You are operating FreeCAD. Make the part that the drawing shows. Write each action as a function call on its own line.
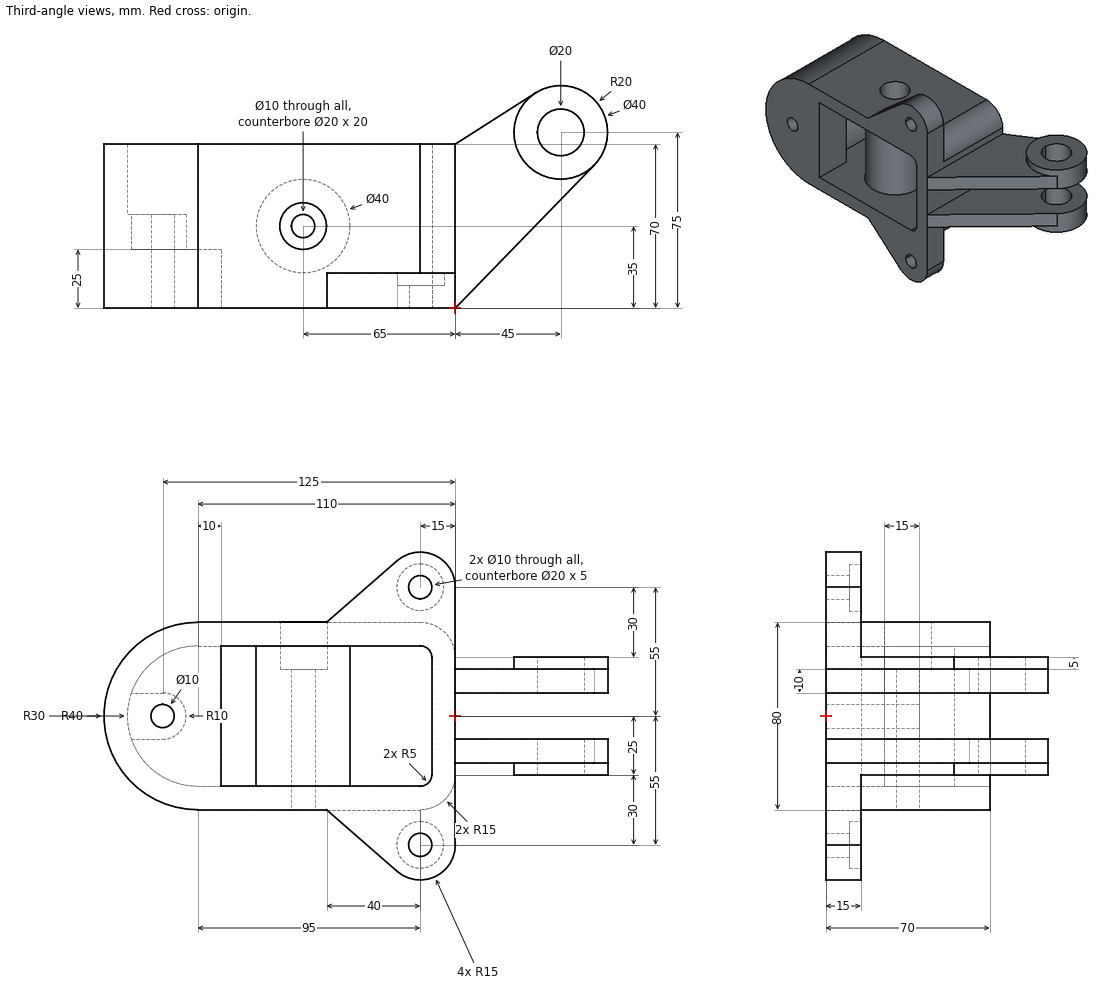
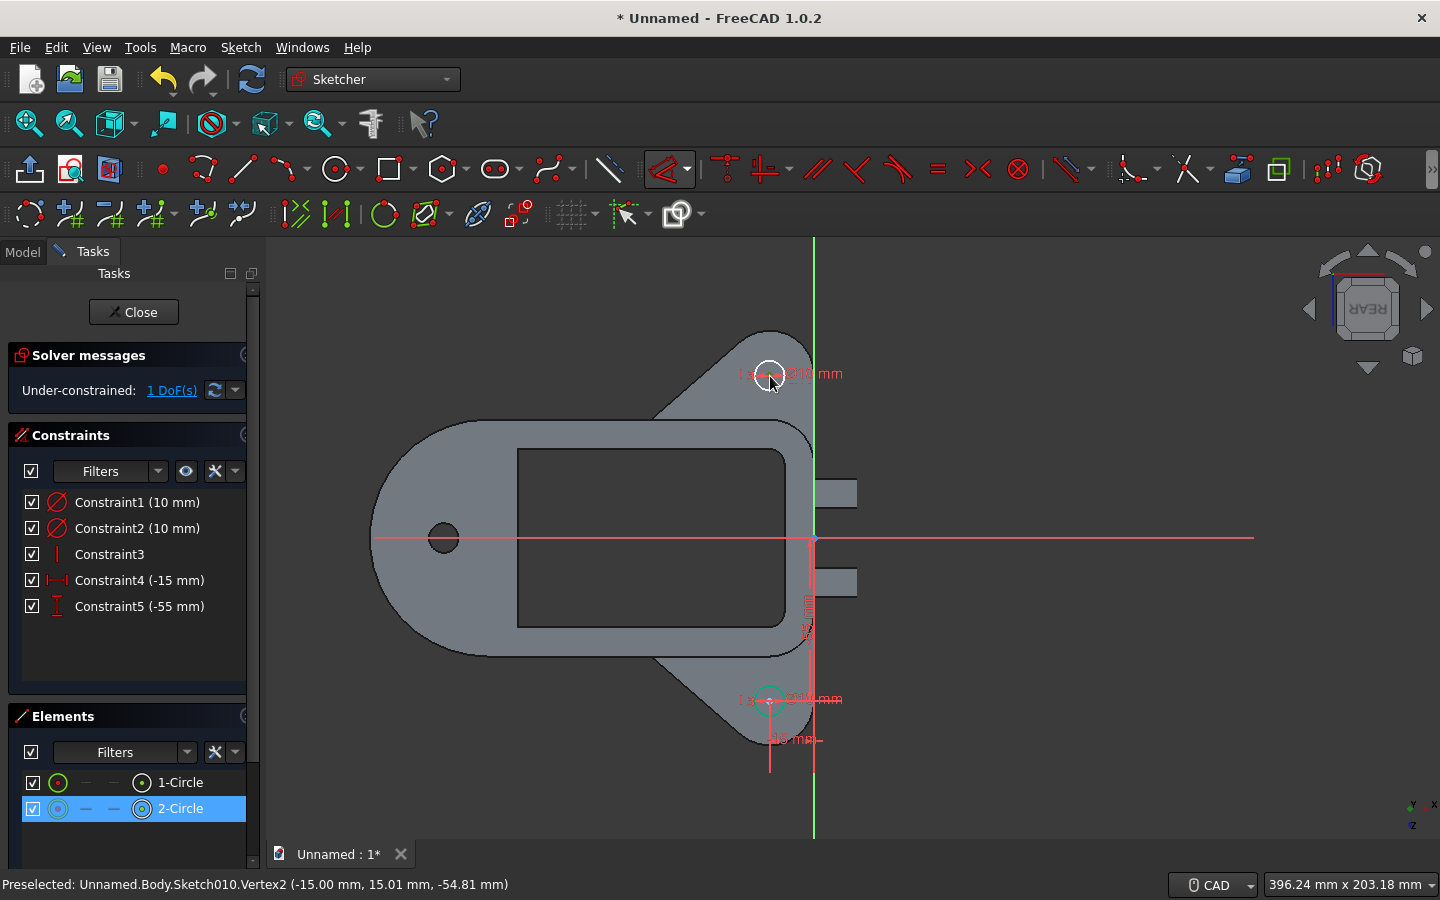
key(i)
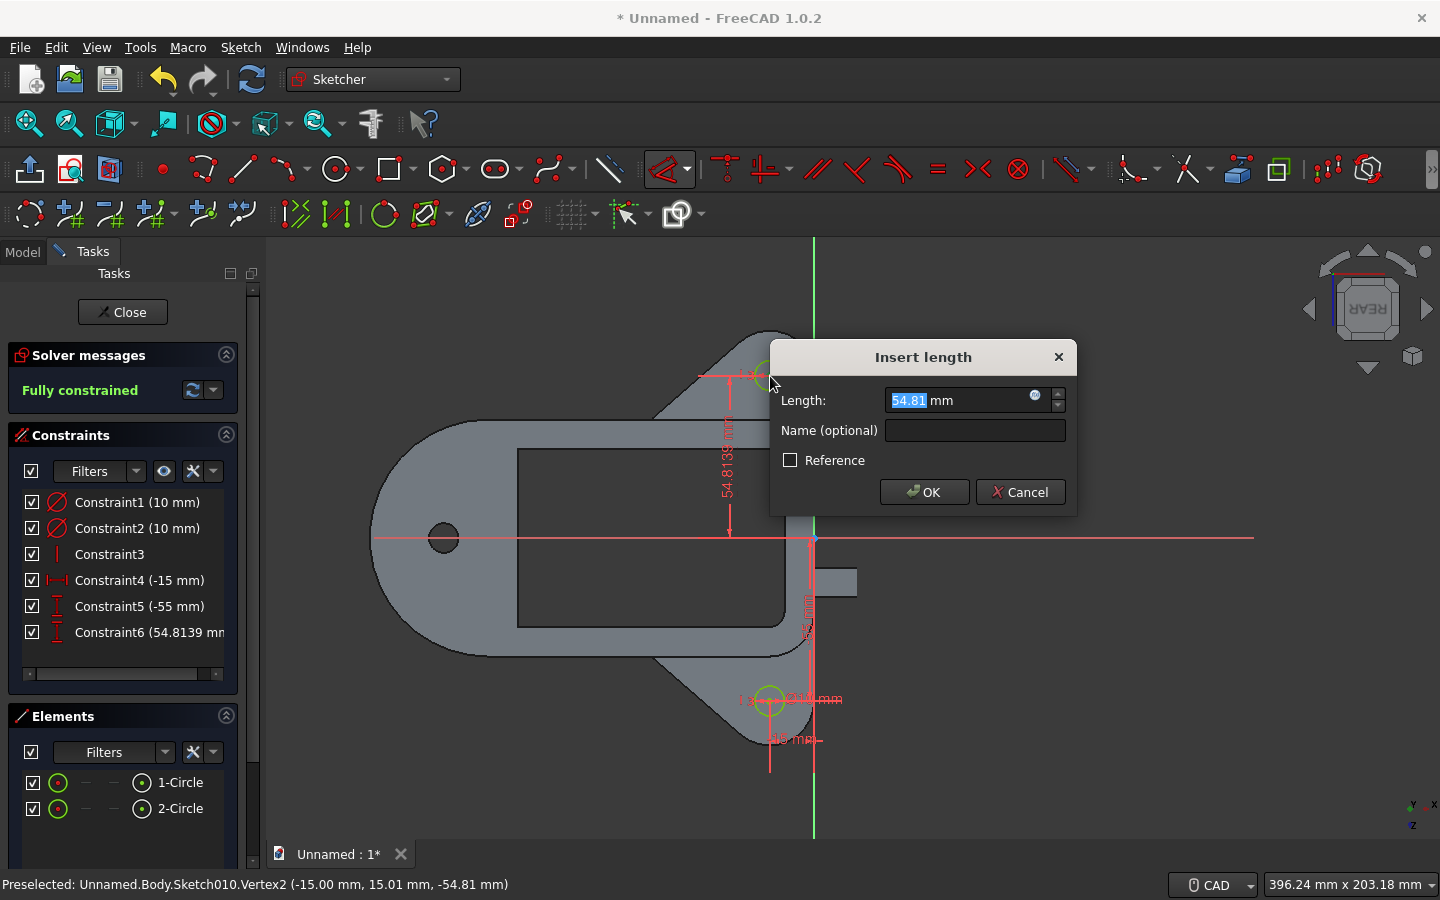
text(55)
key(Return)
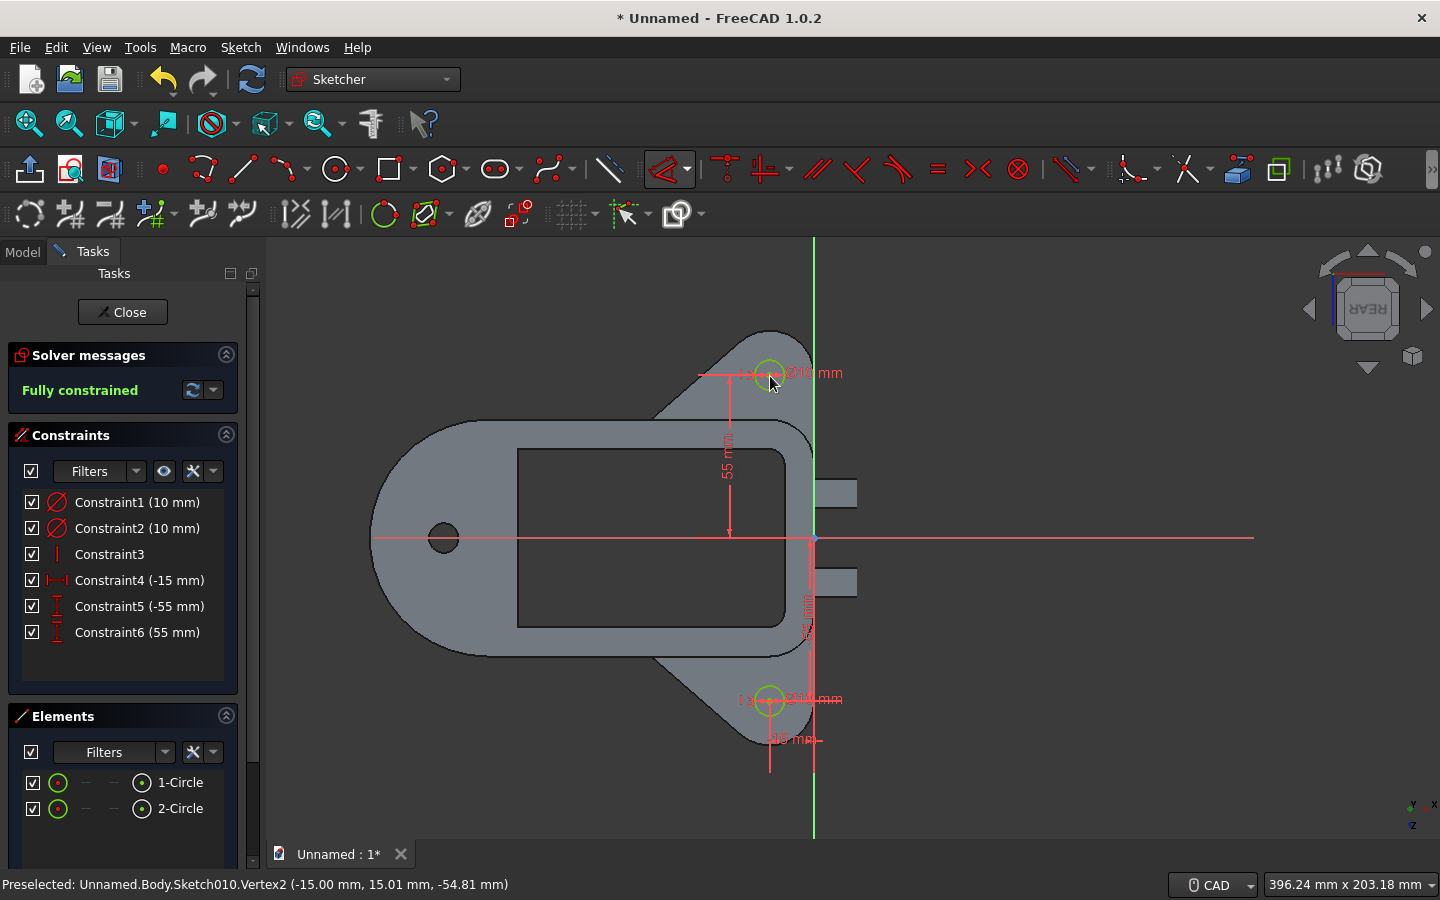
click(123, 312)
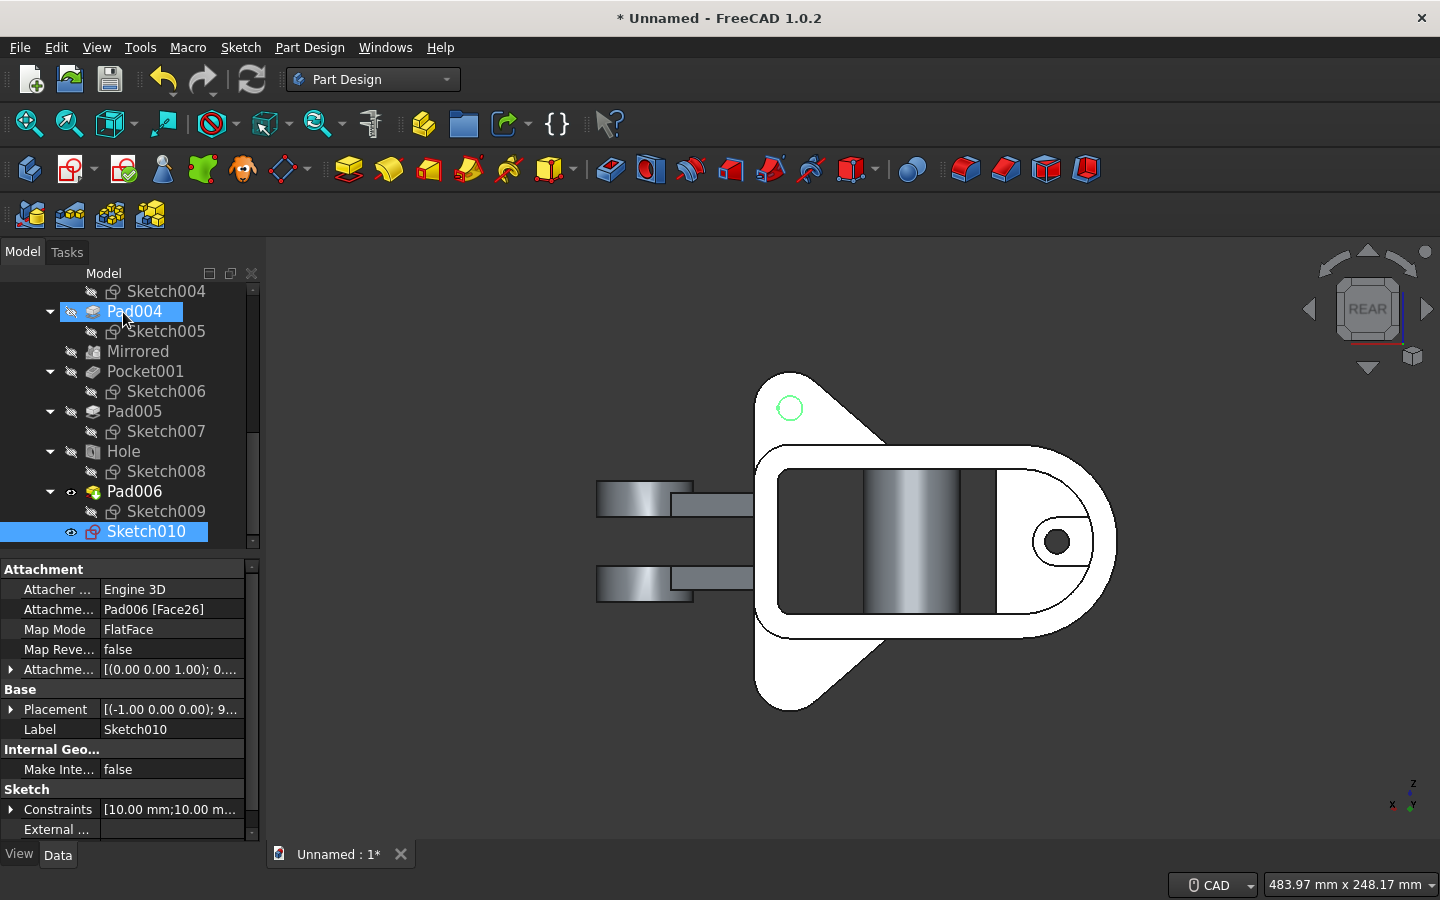
click(652, 170)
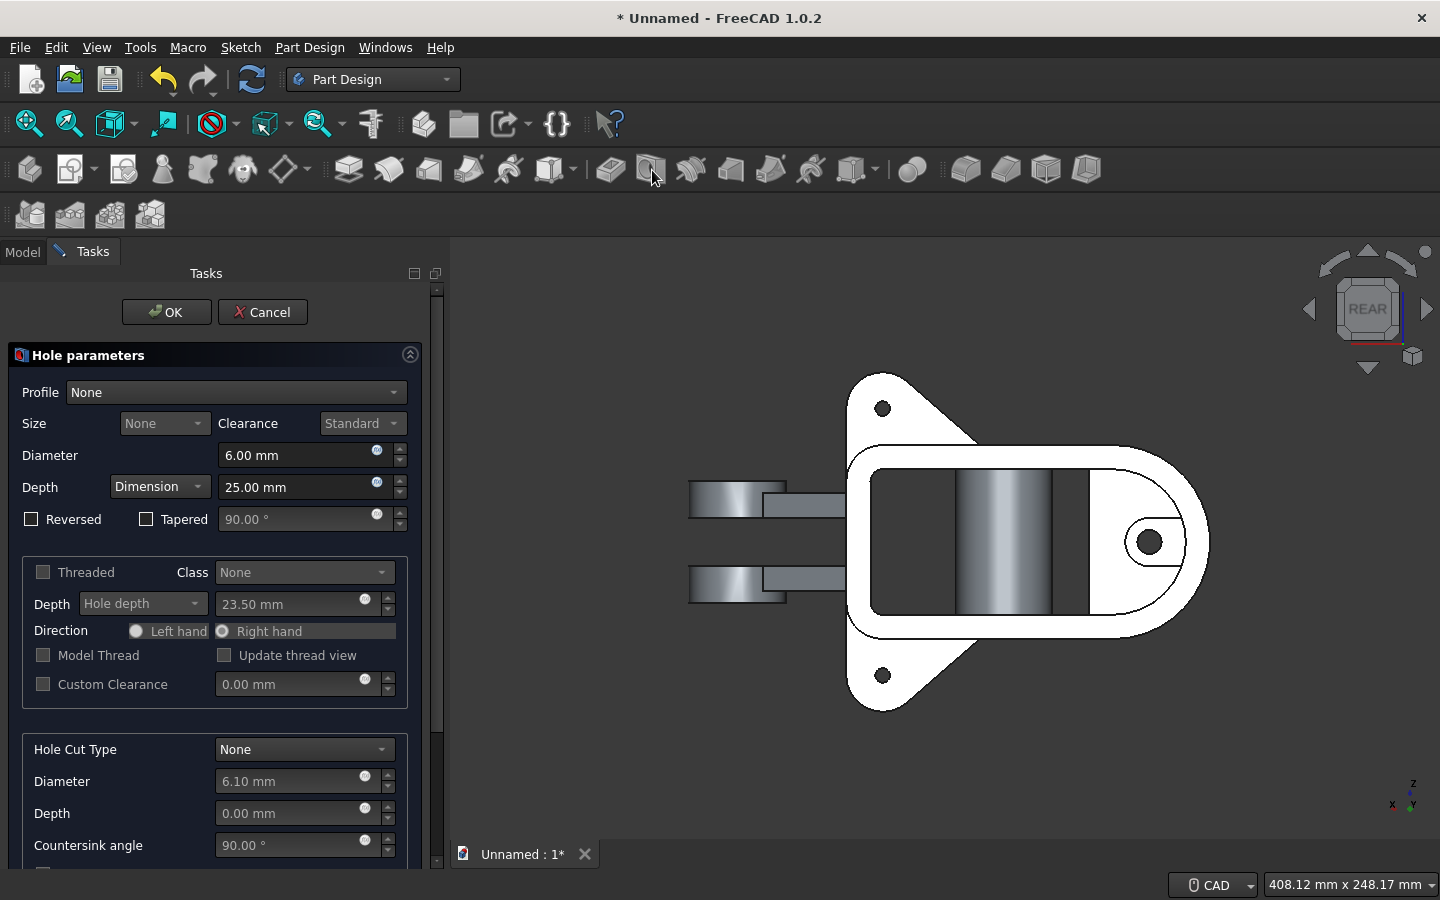
triple_click(305, 455)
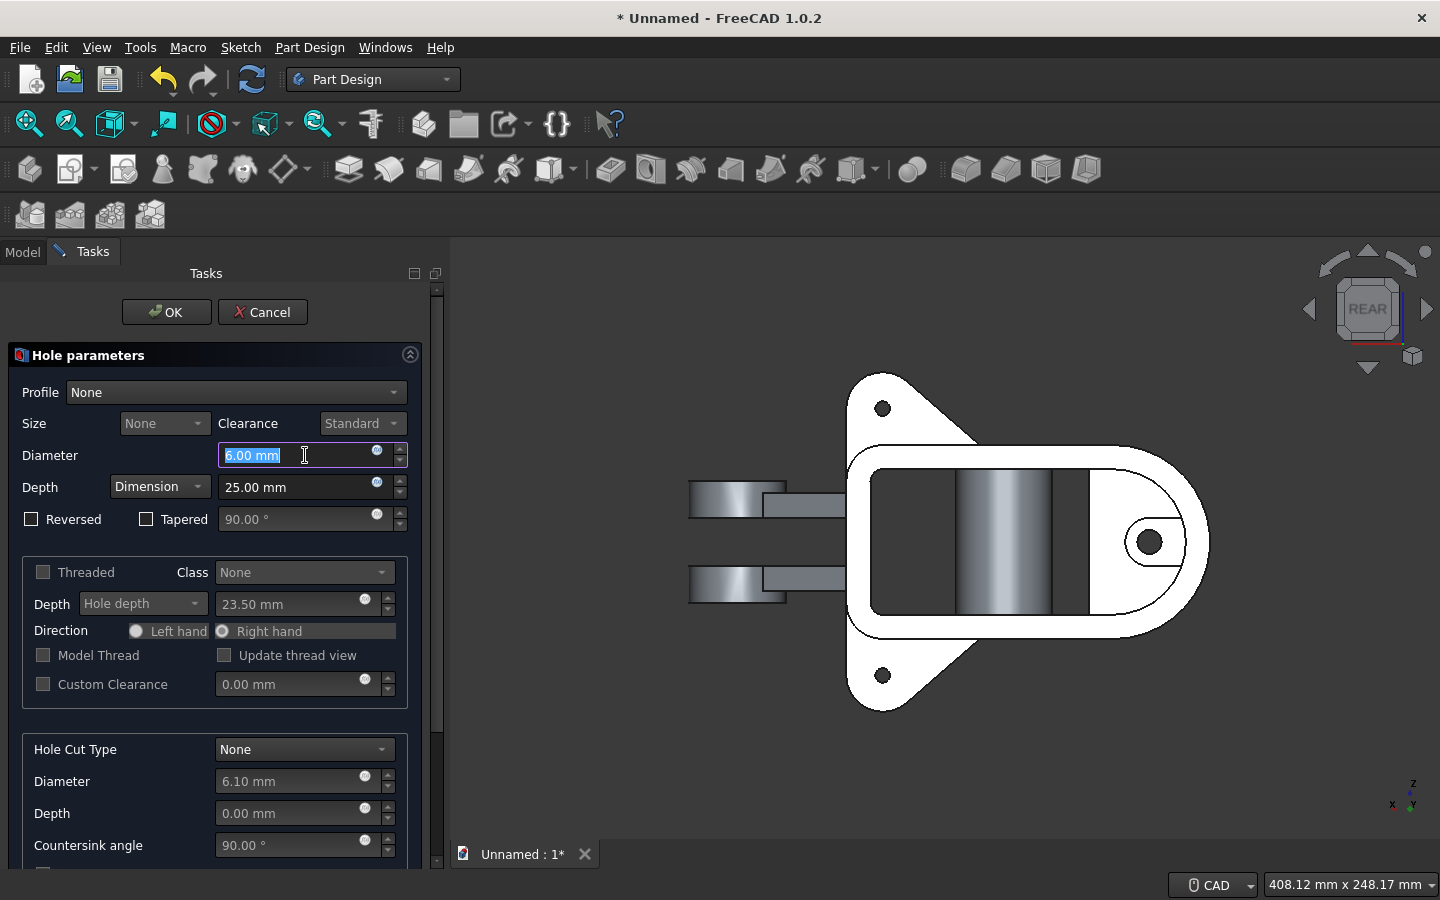
text(10)
key(Tab)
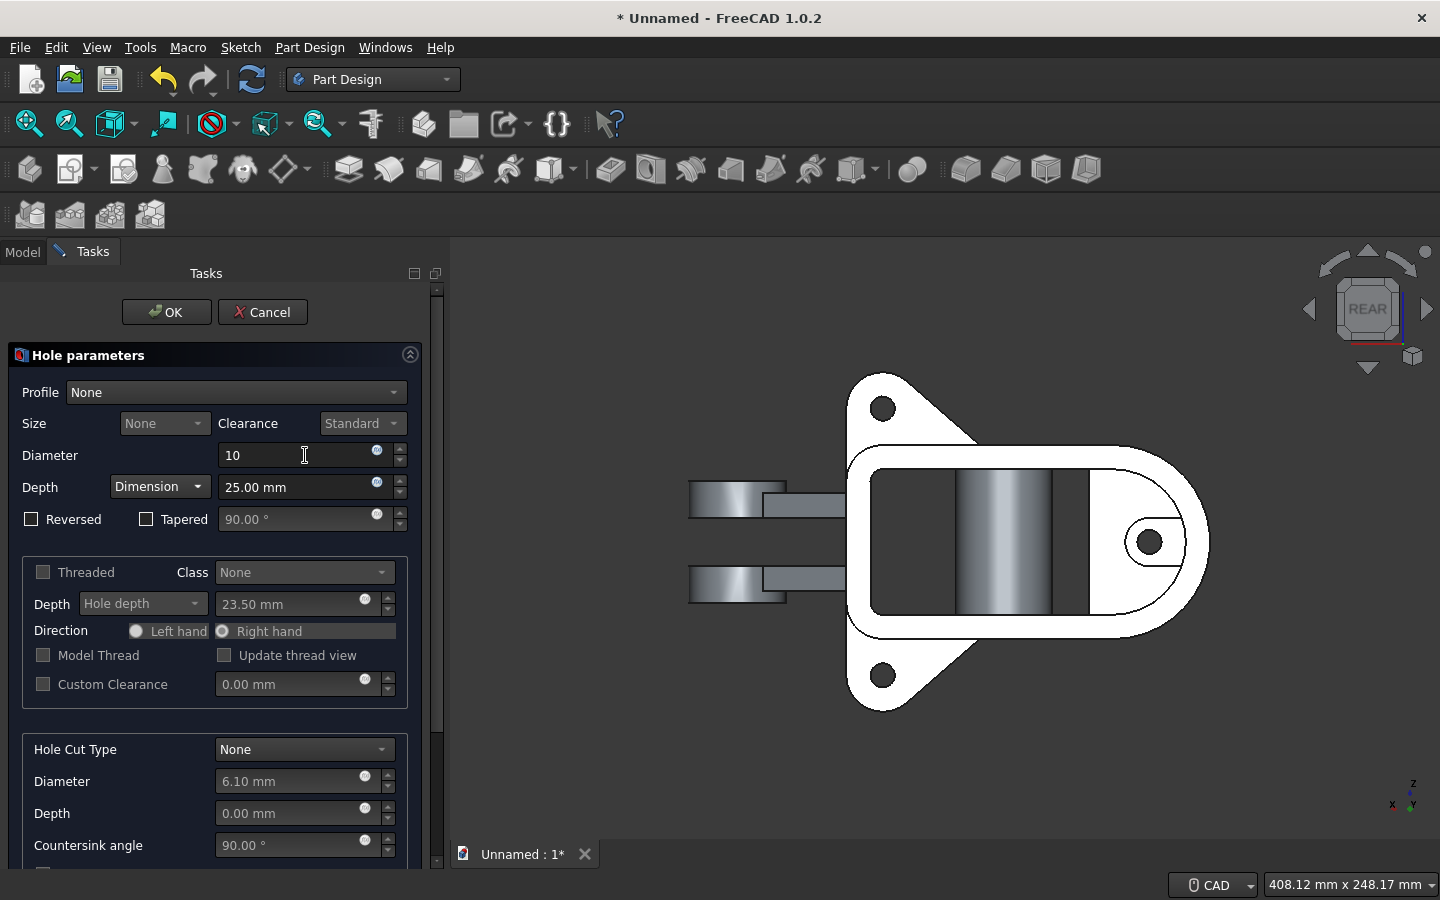
click(161, 486)